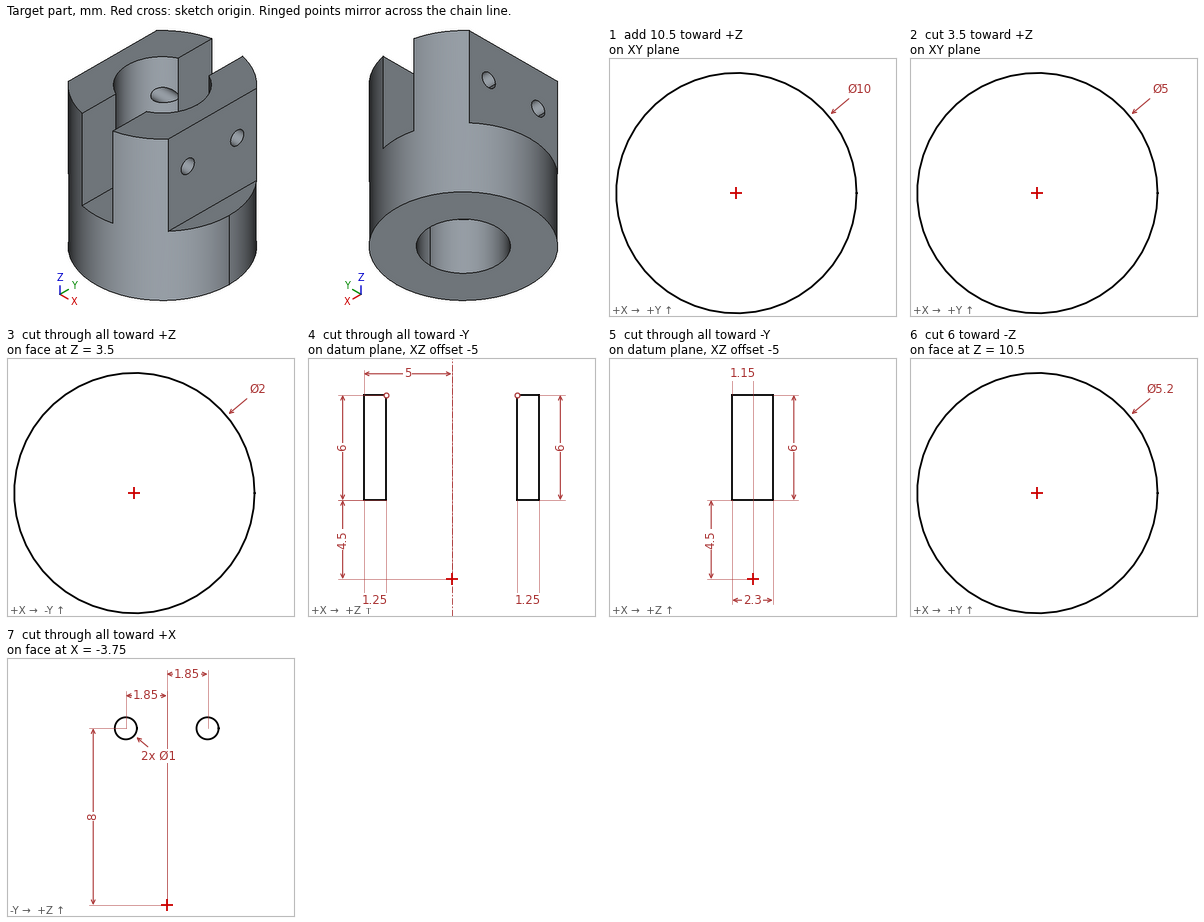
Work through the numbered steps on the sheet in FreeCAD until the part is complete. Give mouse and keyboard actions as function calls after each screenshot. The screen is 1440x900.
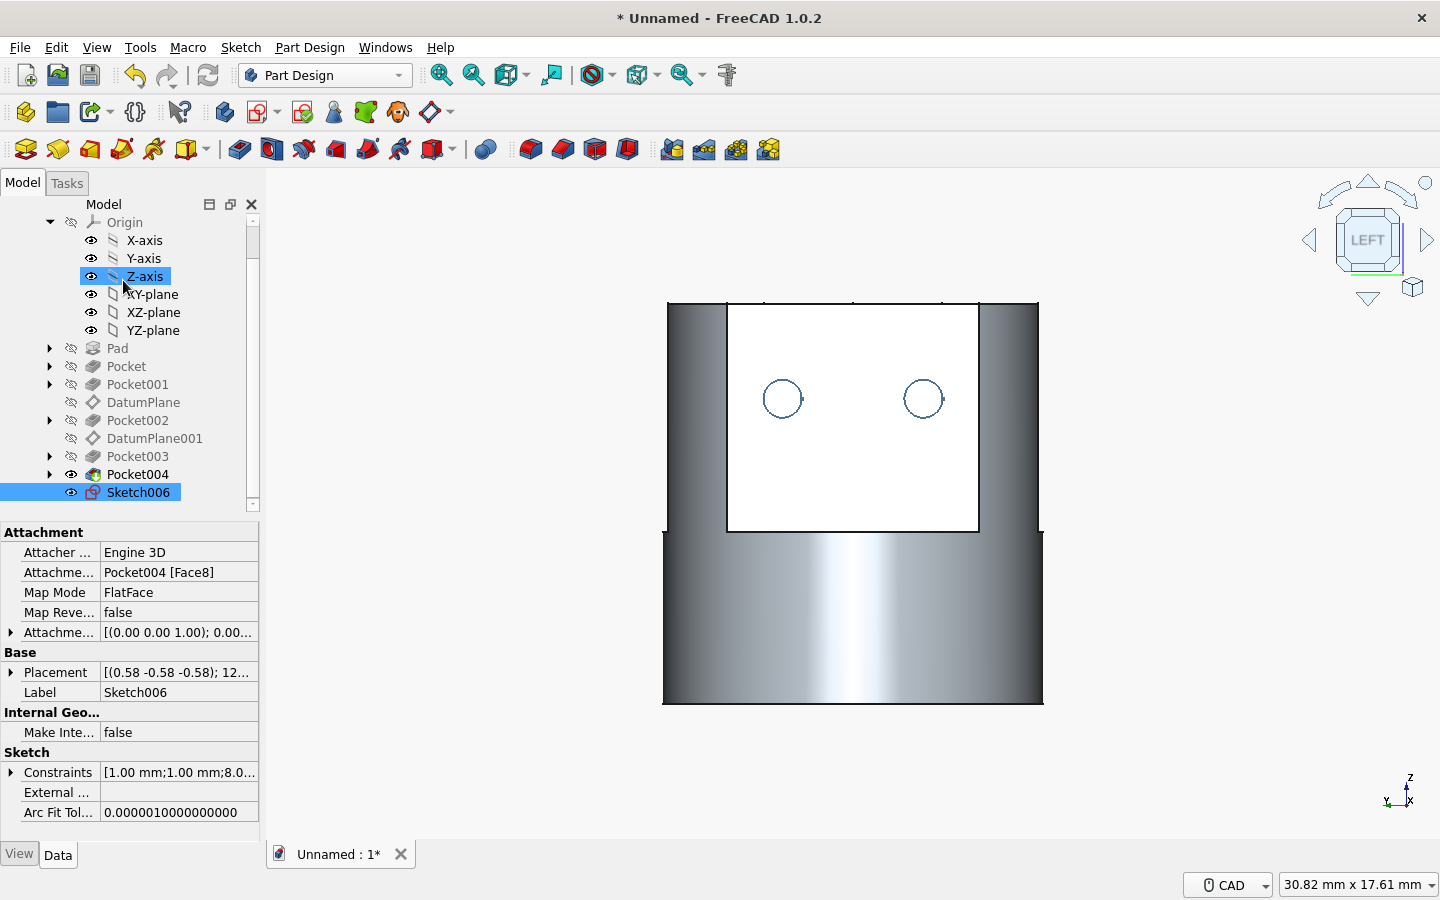
click(240, 150)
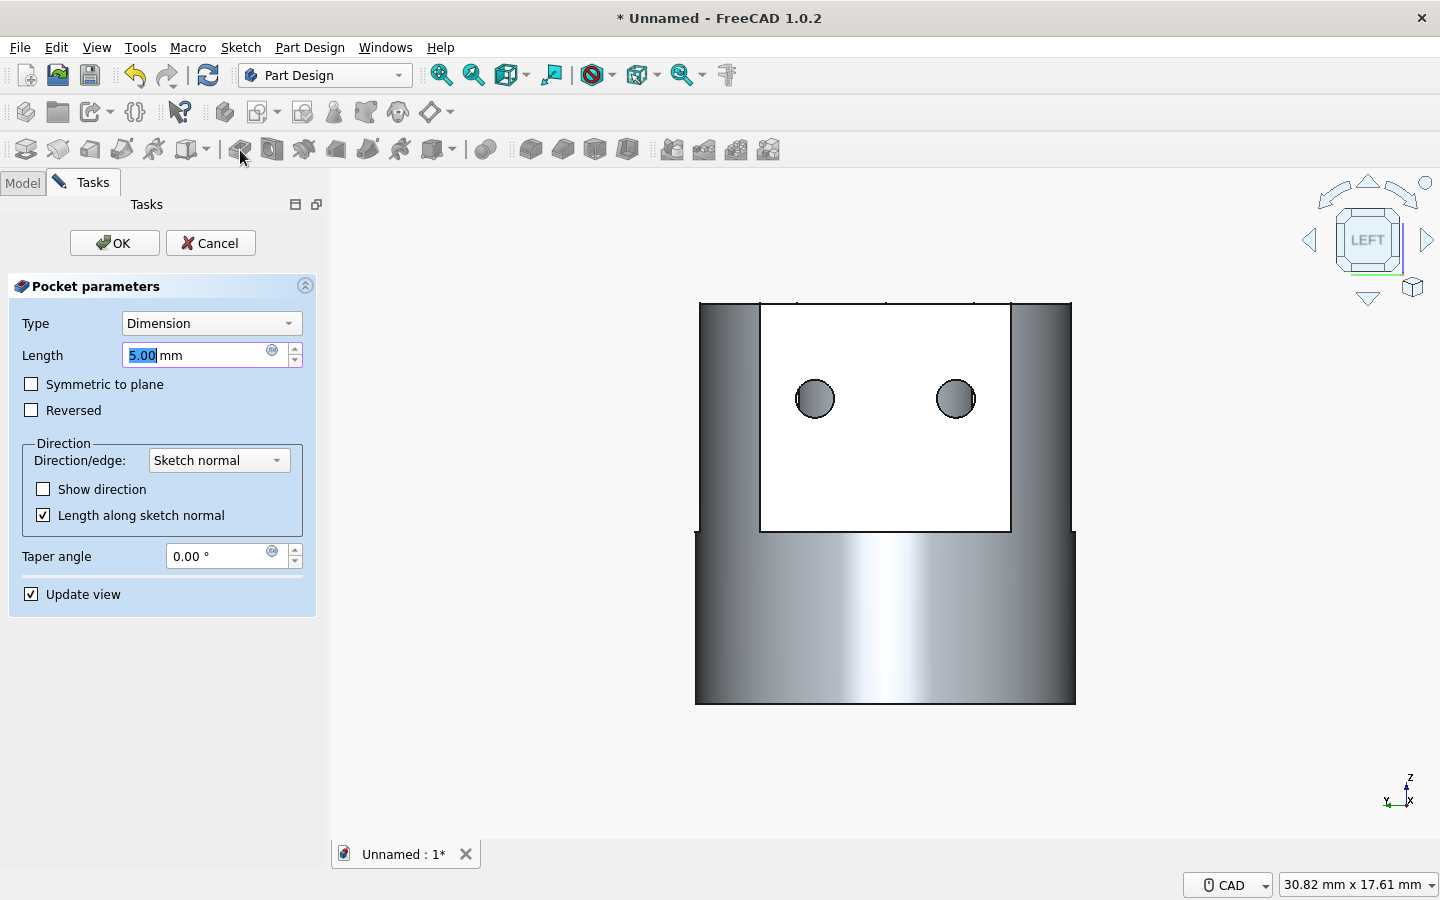
click(212, 324)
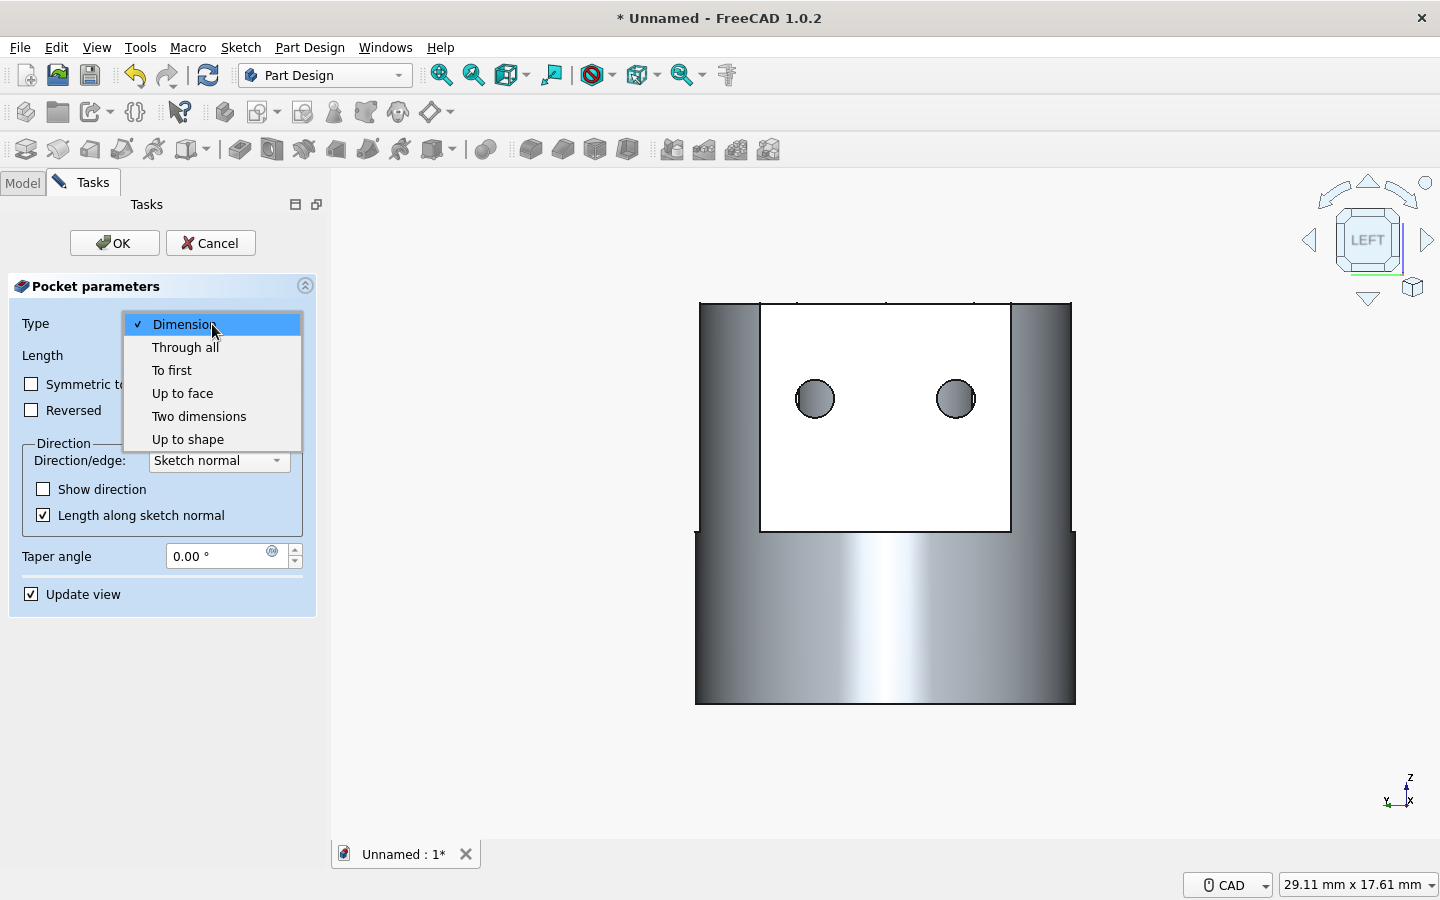
click(212, 348)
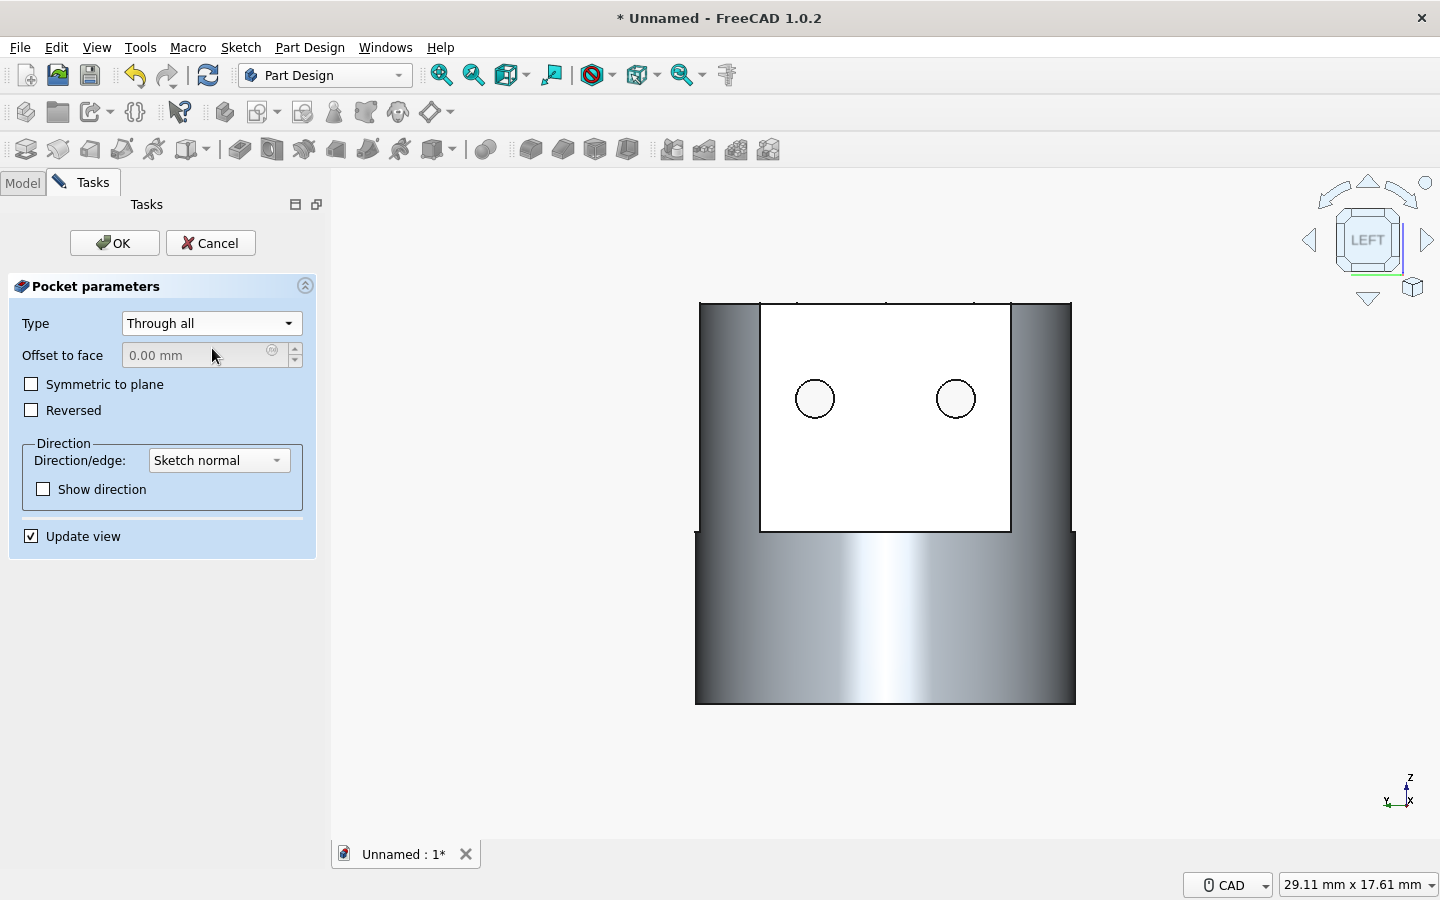
click(115, 243)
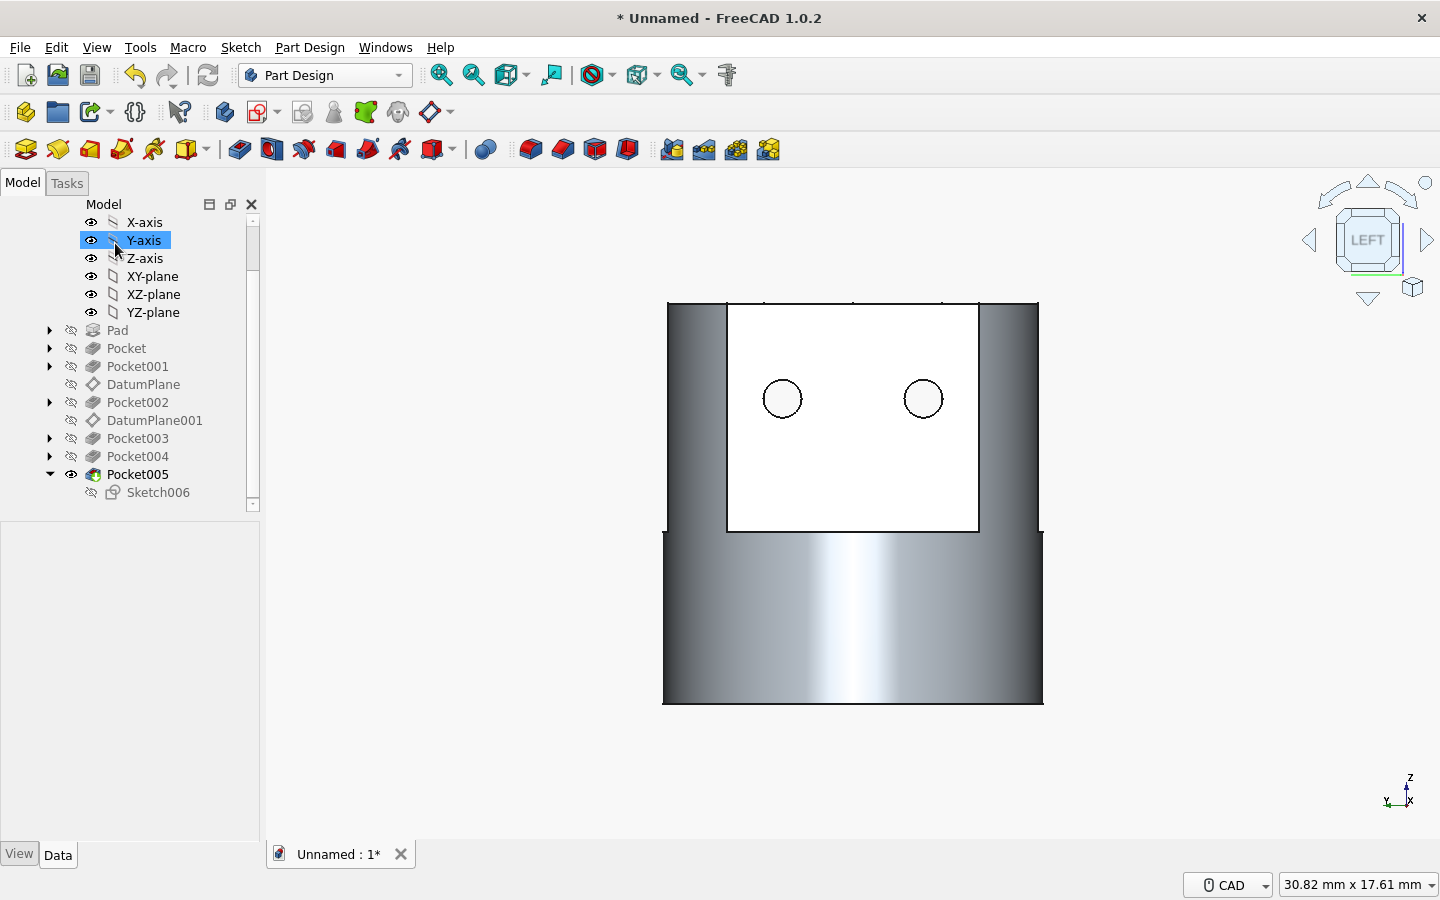
key(0)